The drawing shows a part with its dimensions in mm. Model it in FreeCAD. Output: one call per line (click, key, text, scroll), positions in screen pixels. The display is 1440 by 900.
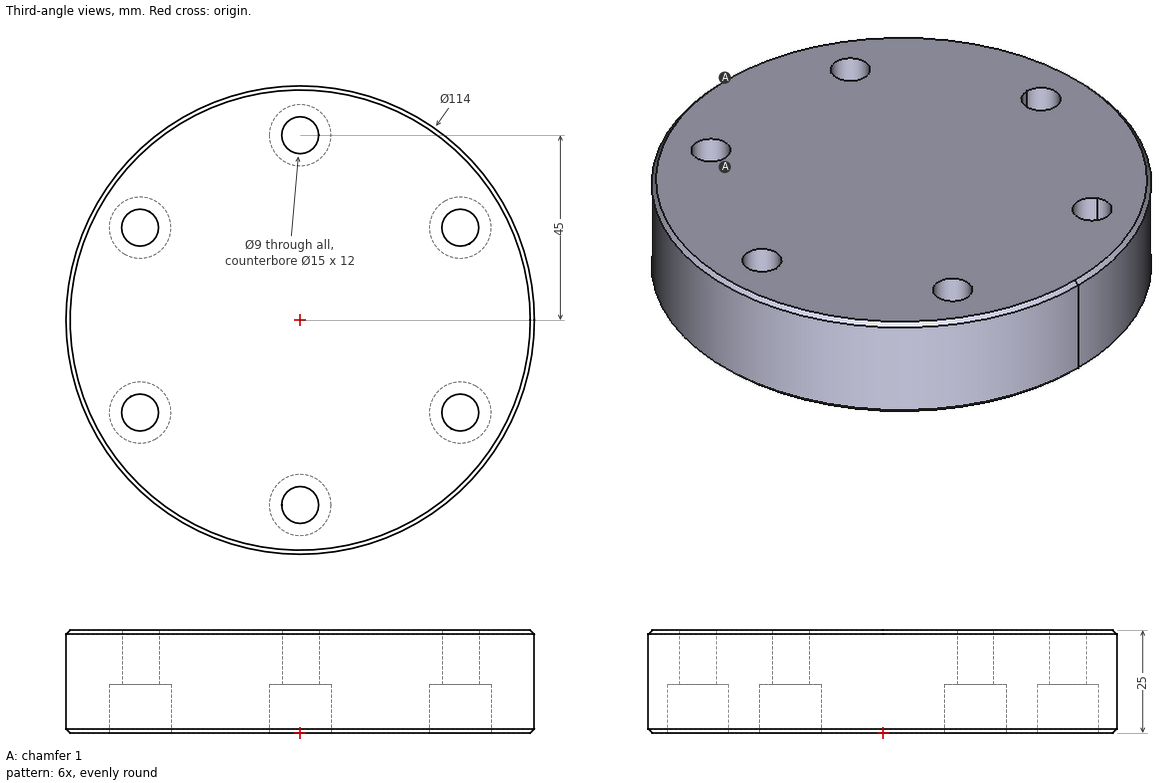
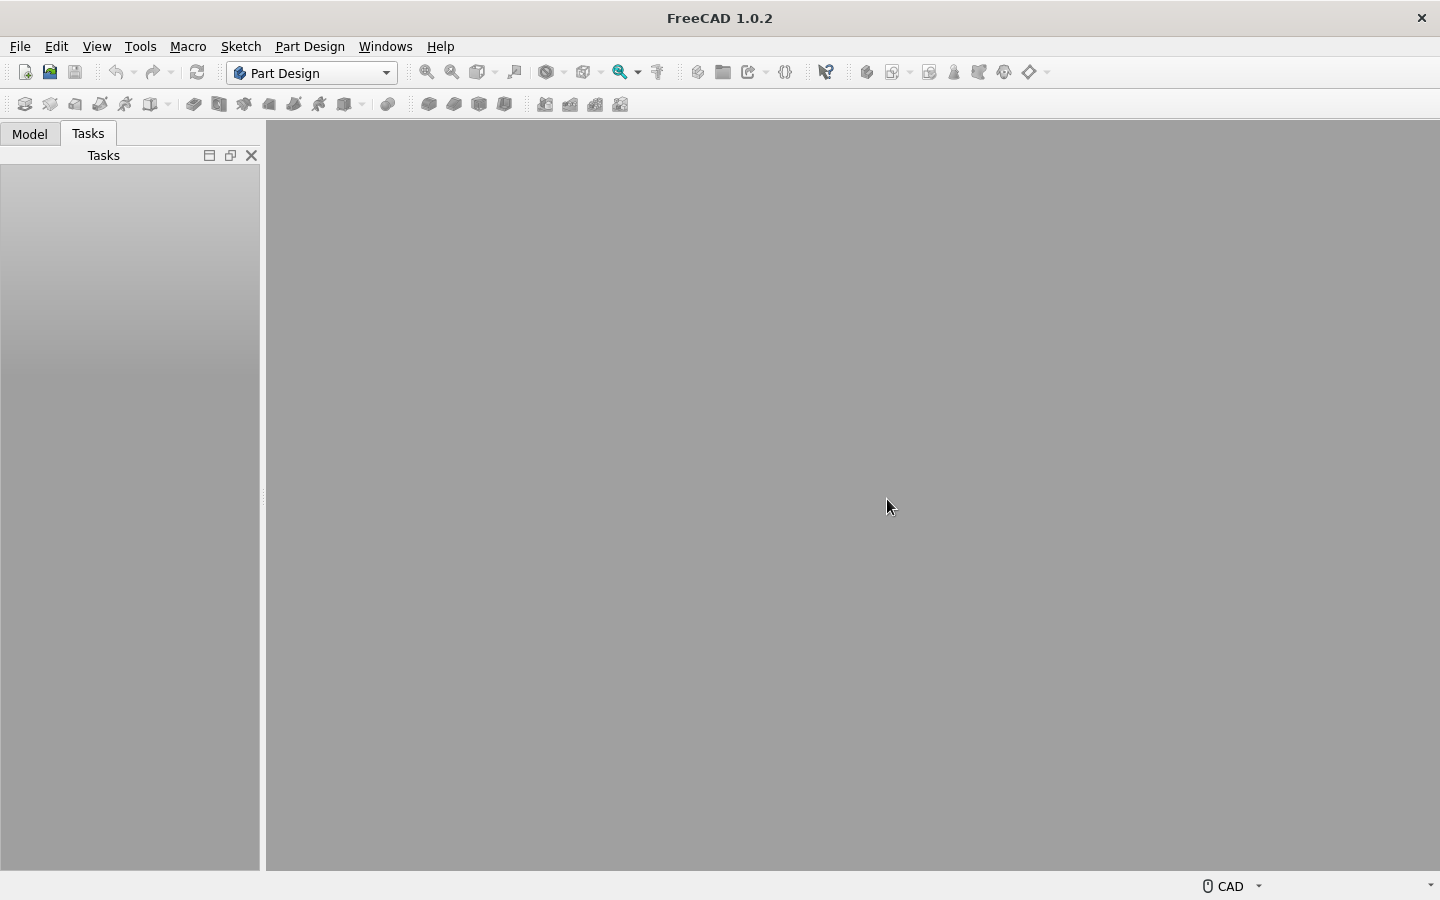
click(25, 72)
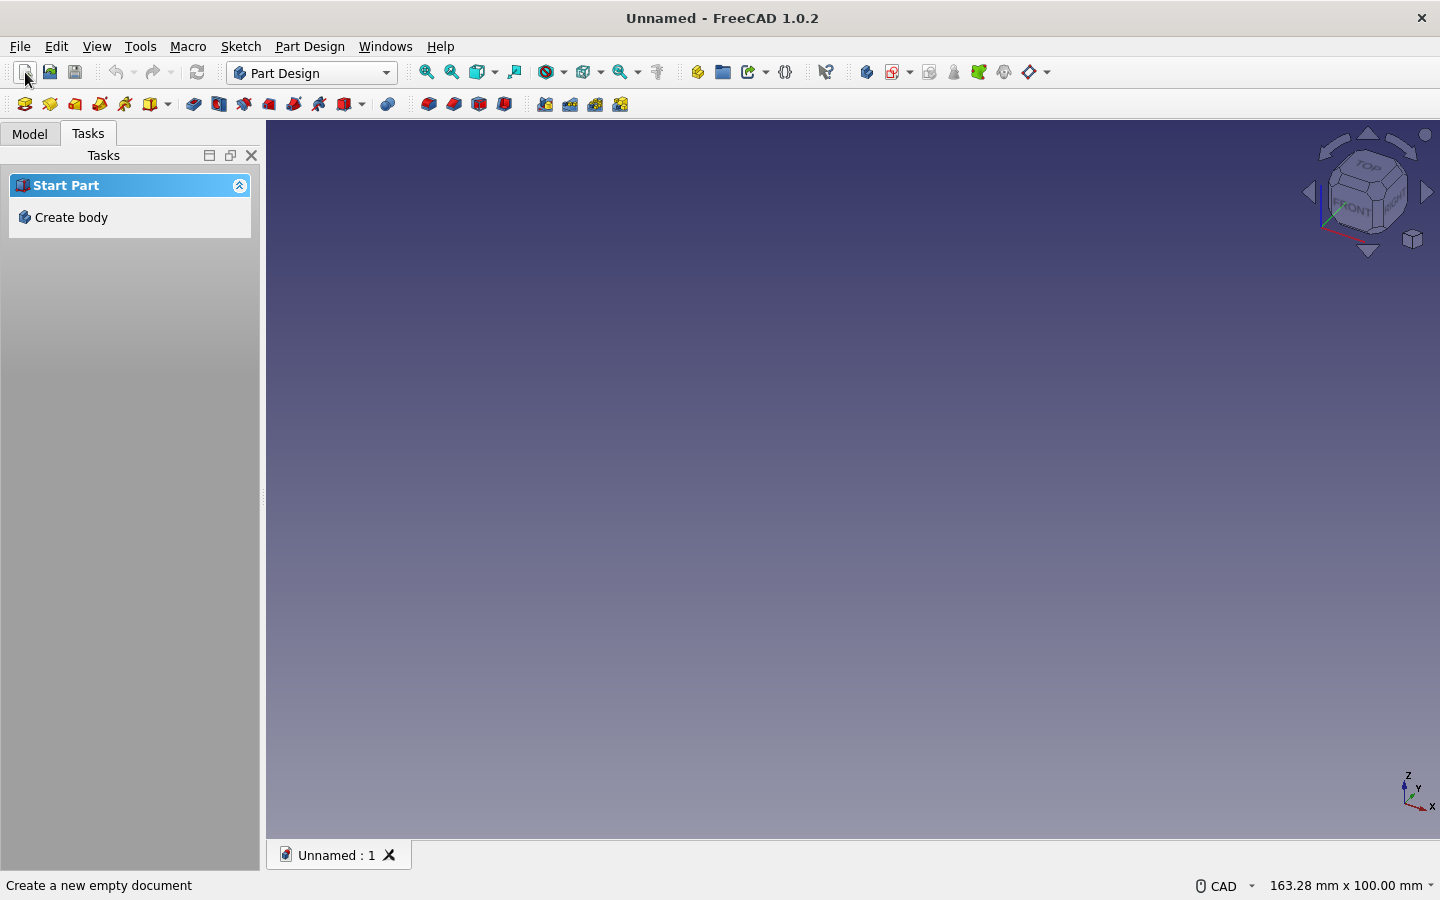
click(892, 72)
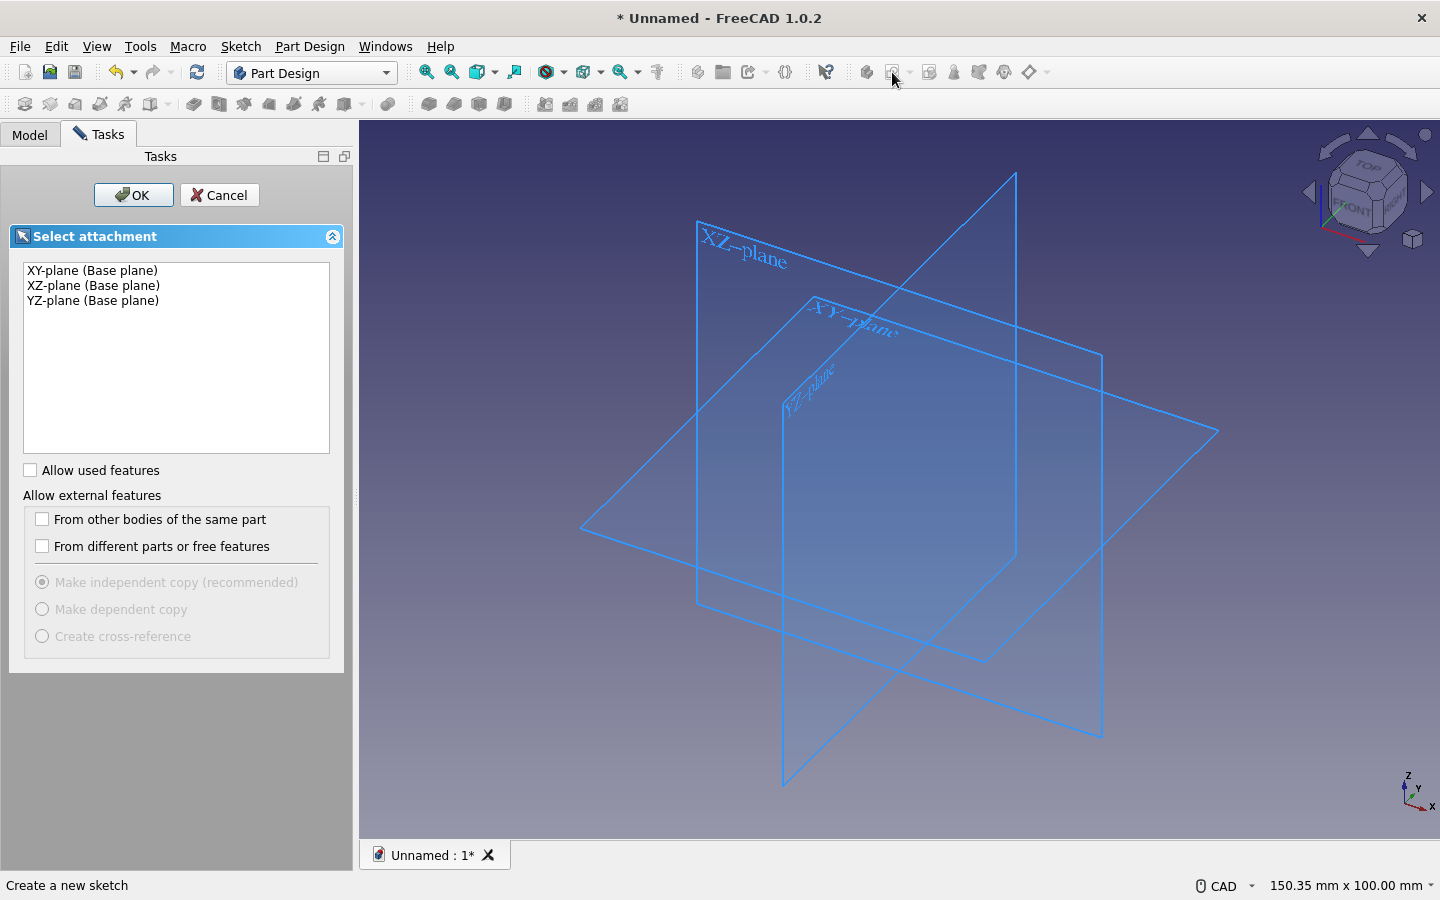
click(84, 270)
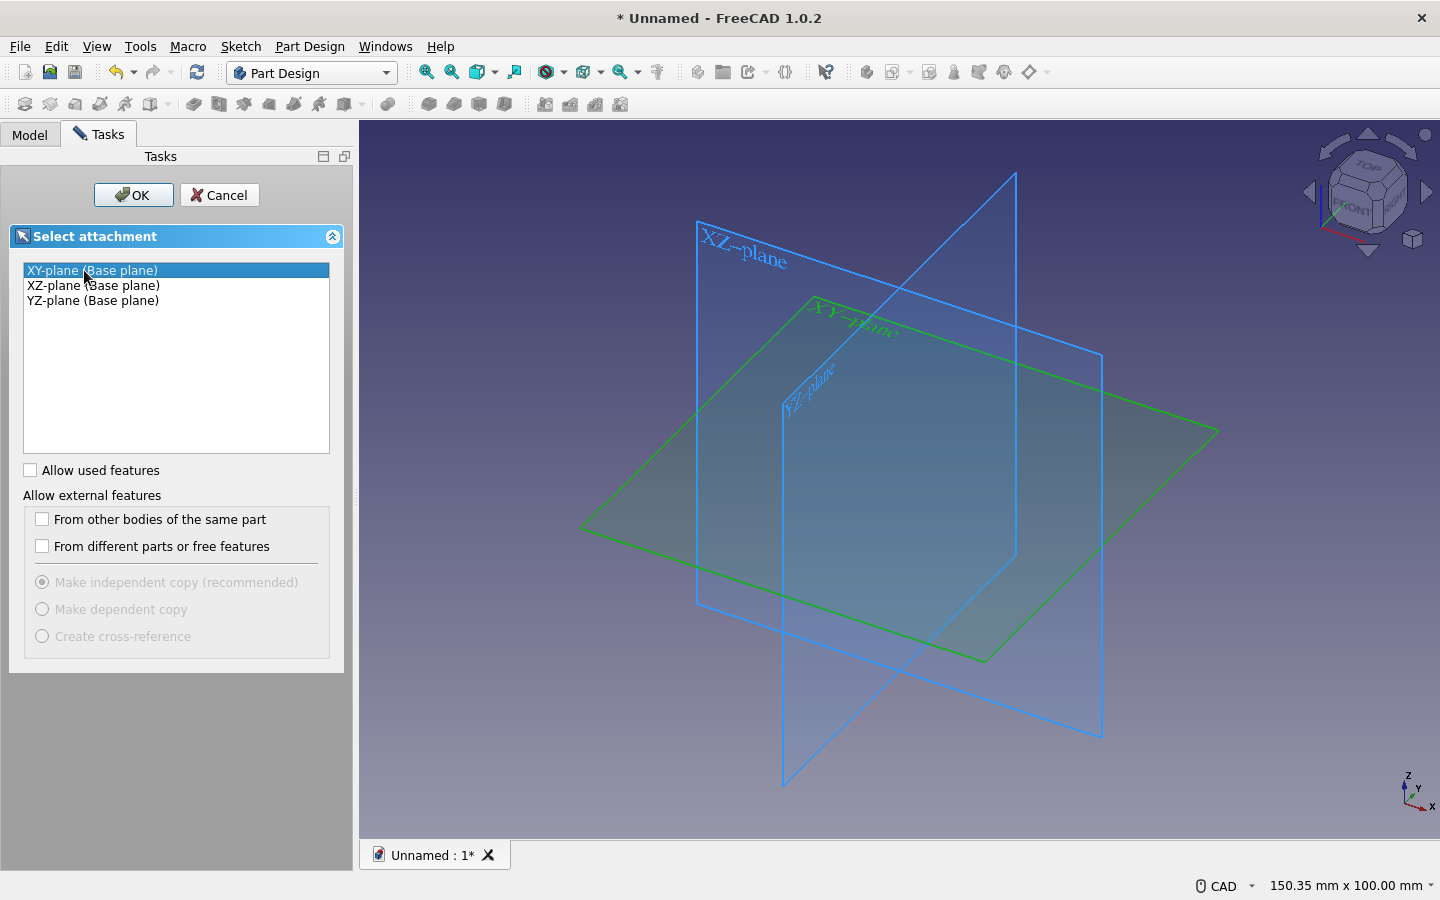
click(134, 195)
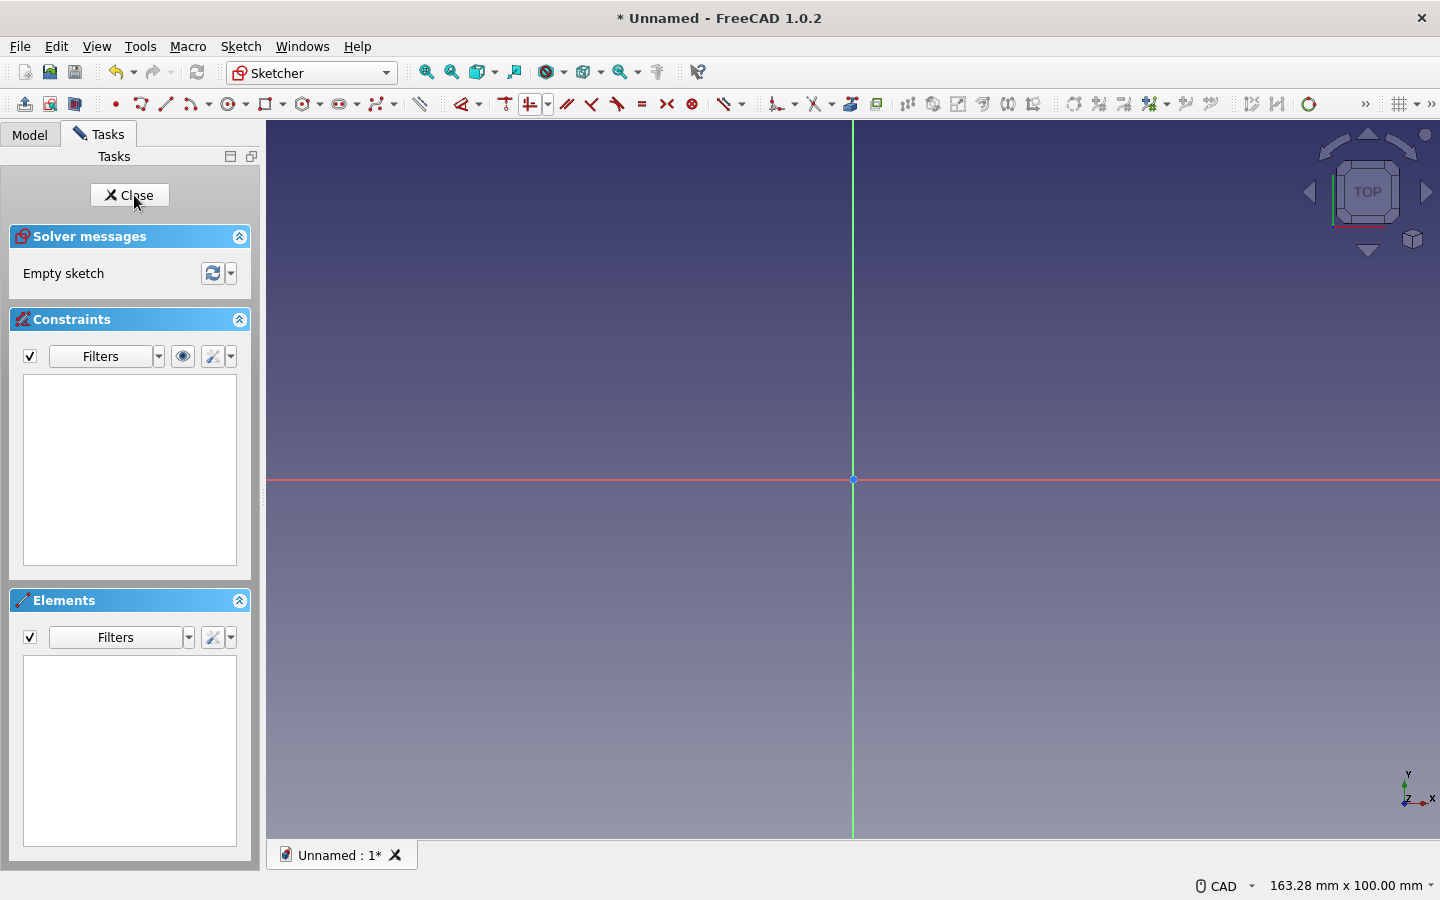
scroll(701, 479, down, 3)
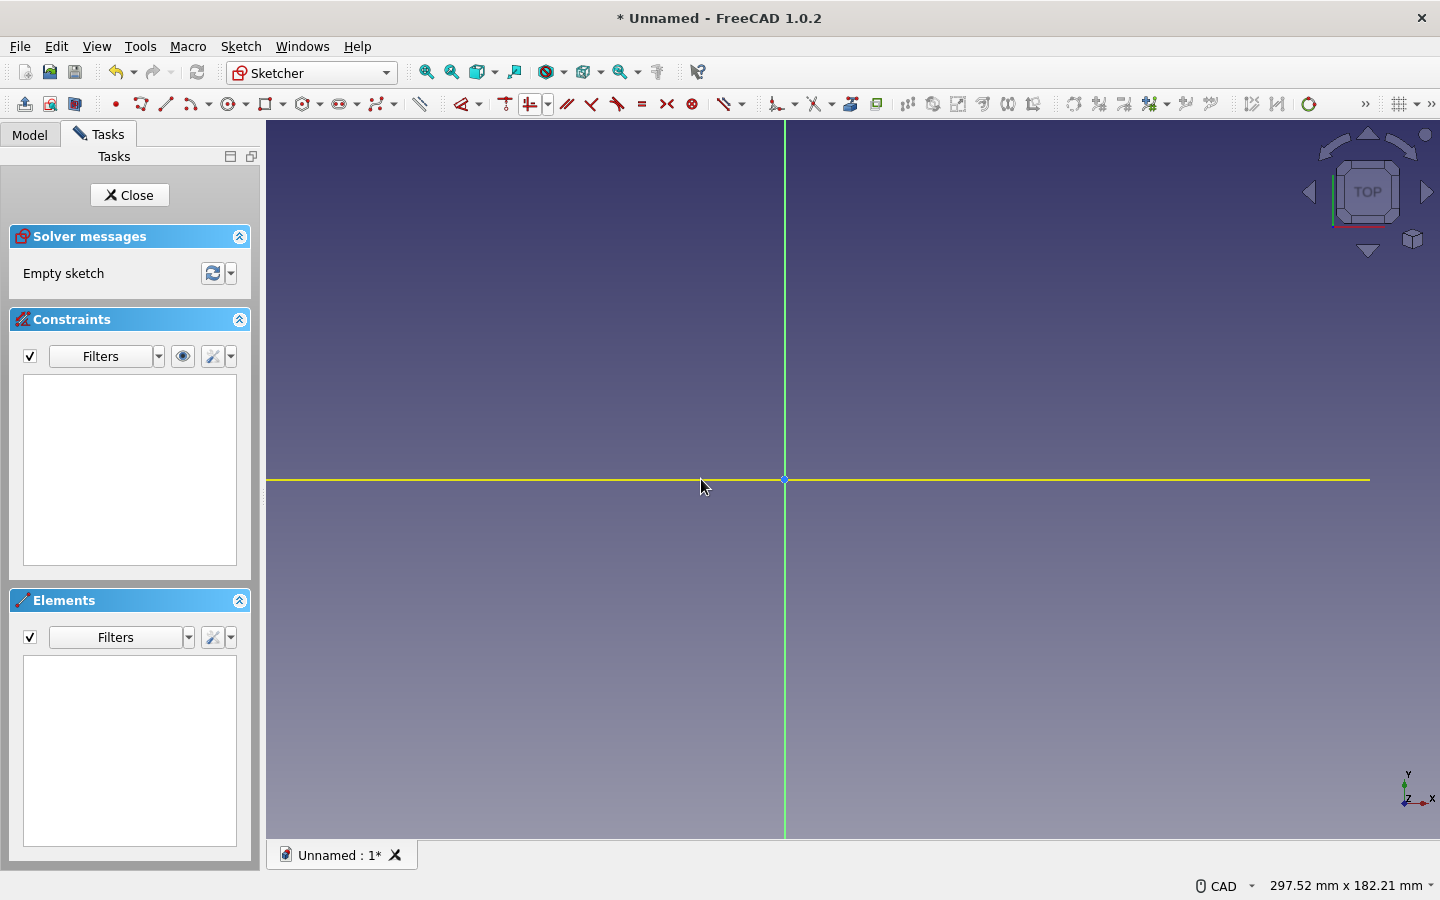
click(228, 104)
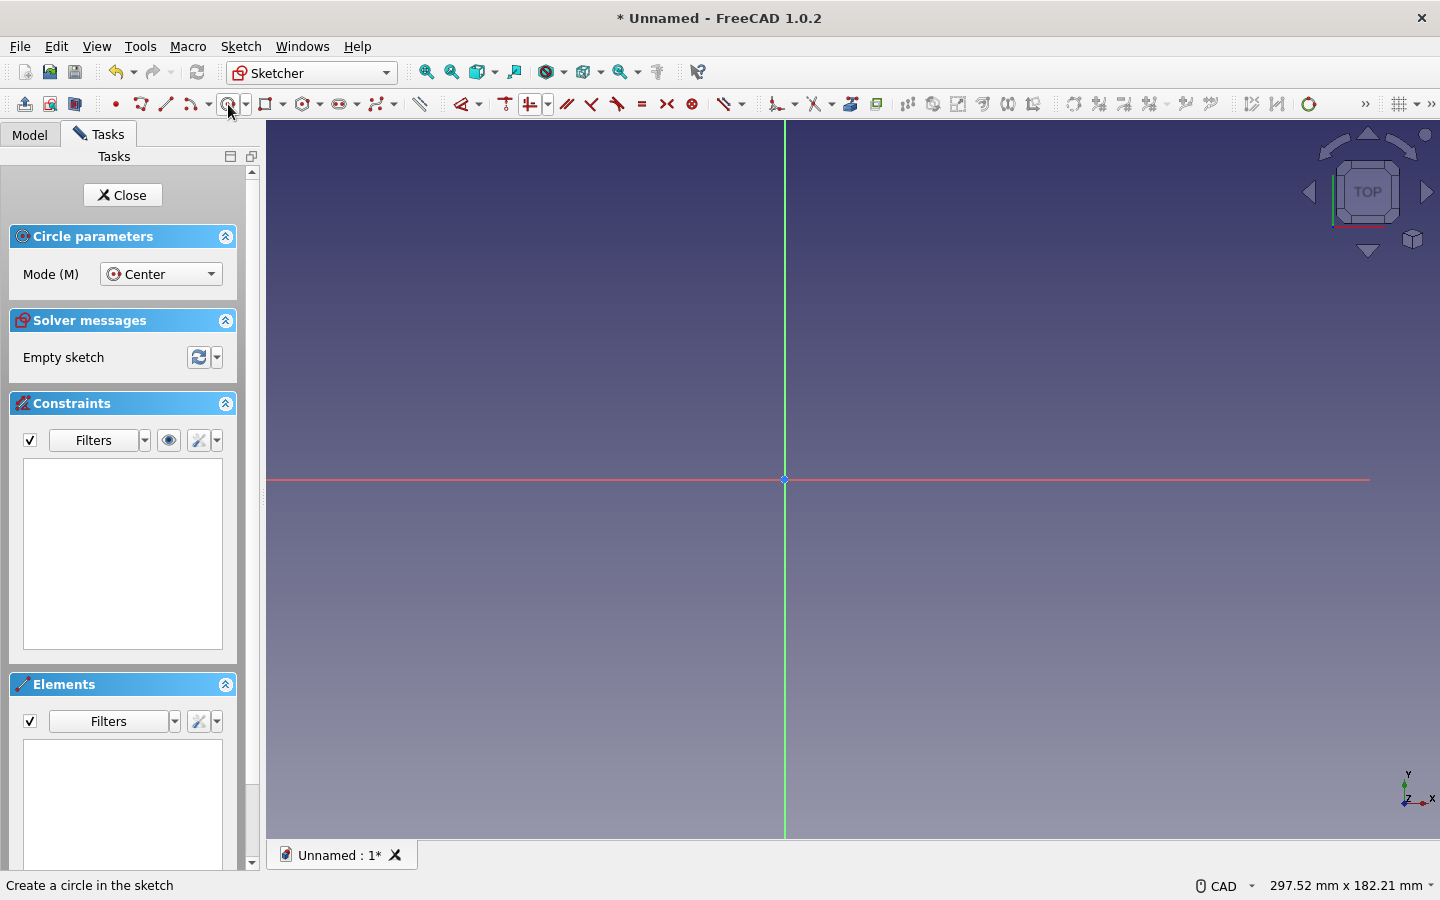
click(785, 480)
move(944, 320)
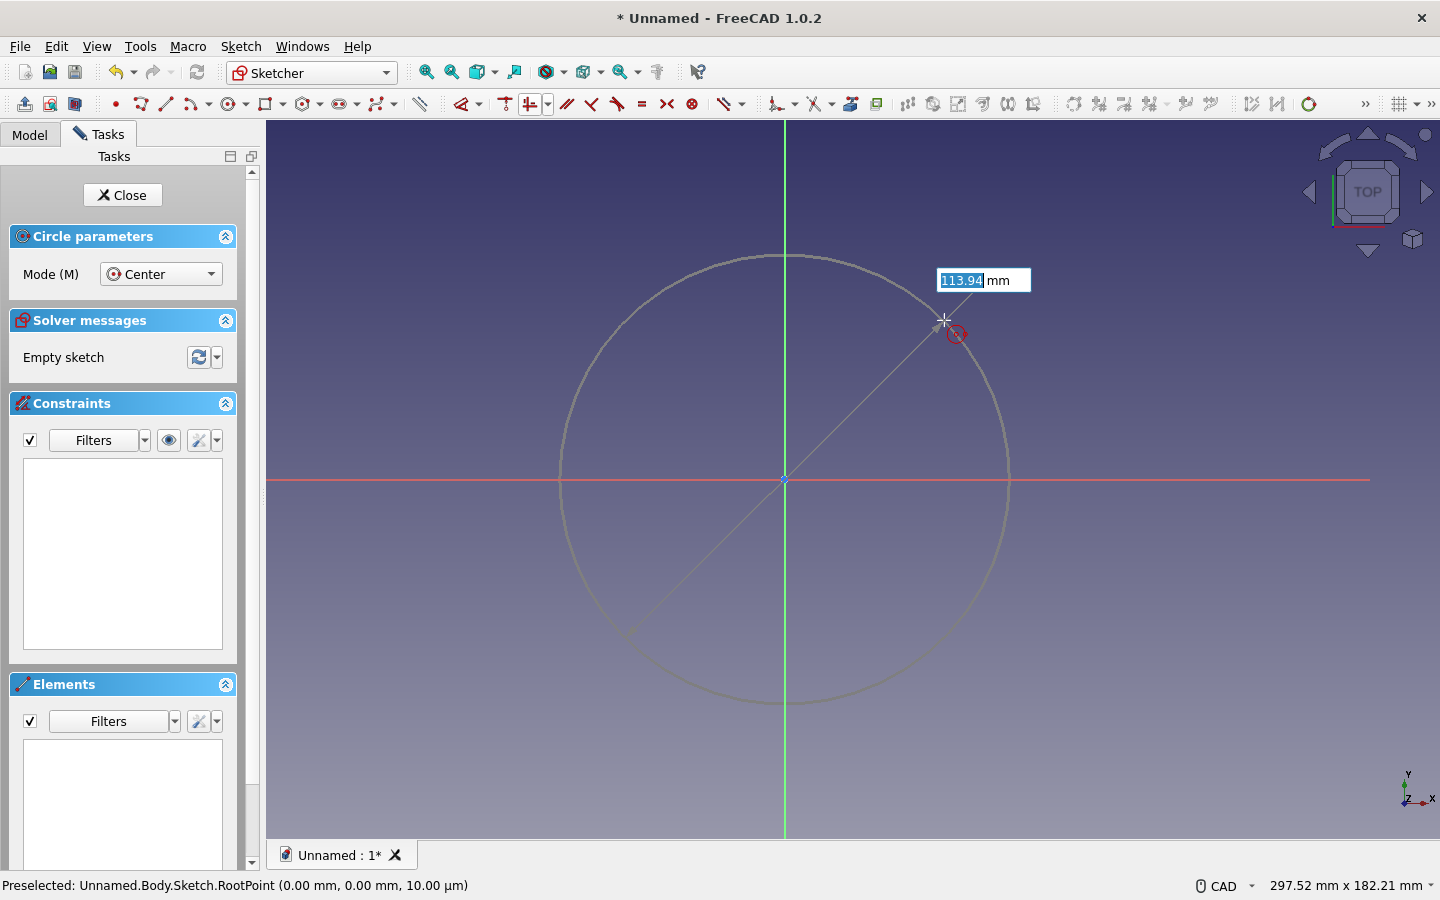
text(114)
key(Return)
key(Escape)